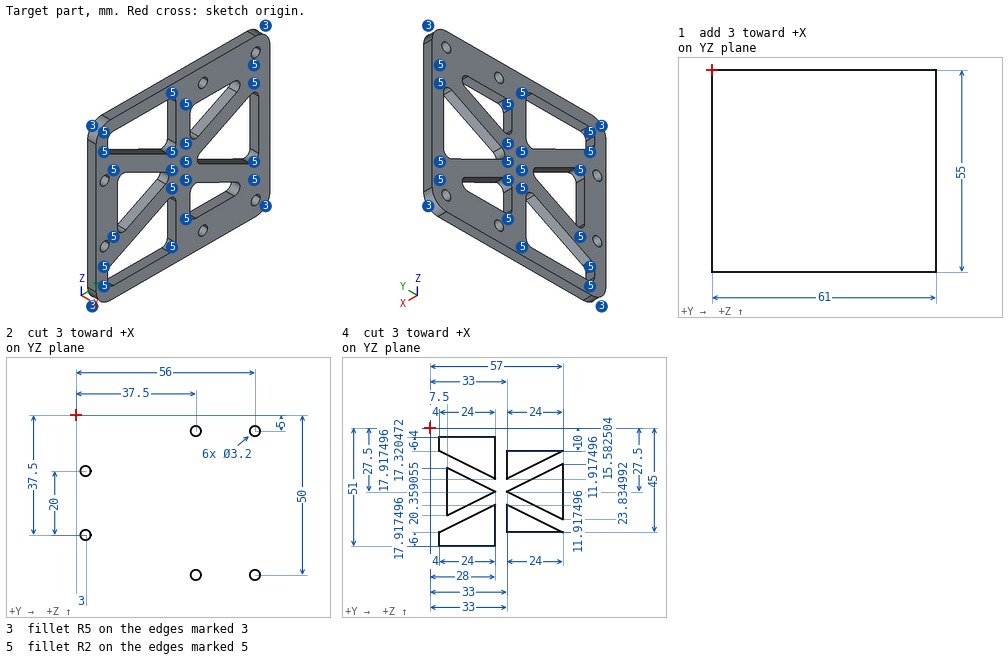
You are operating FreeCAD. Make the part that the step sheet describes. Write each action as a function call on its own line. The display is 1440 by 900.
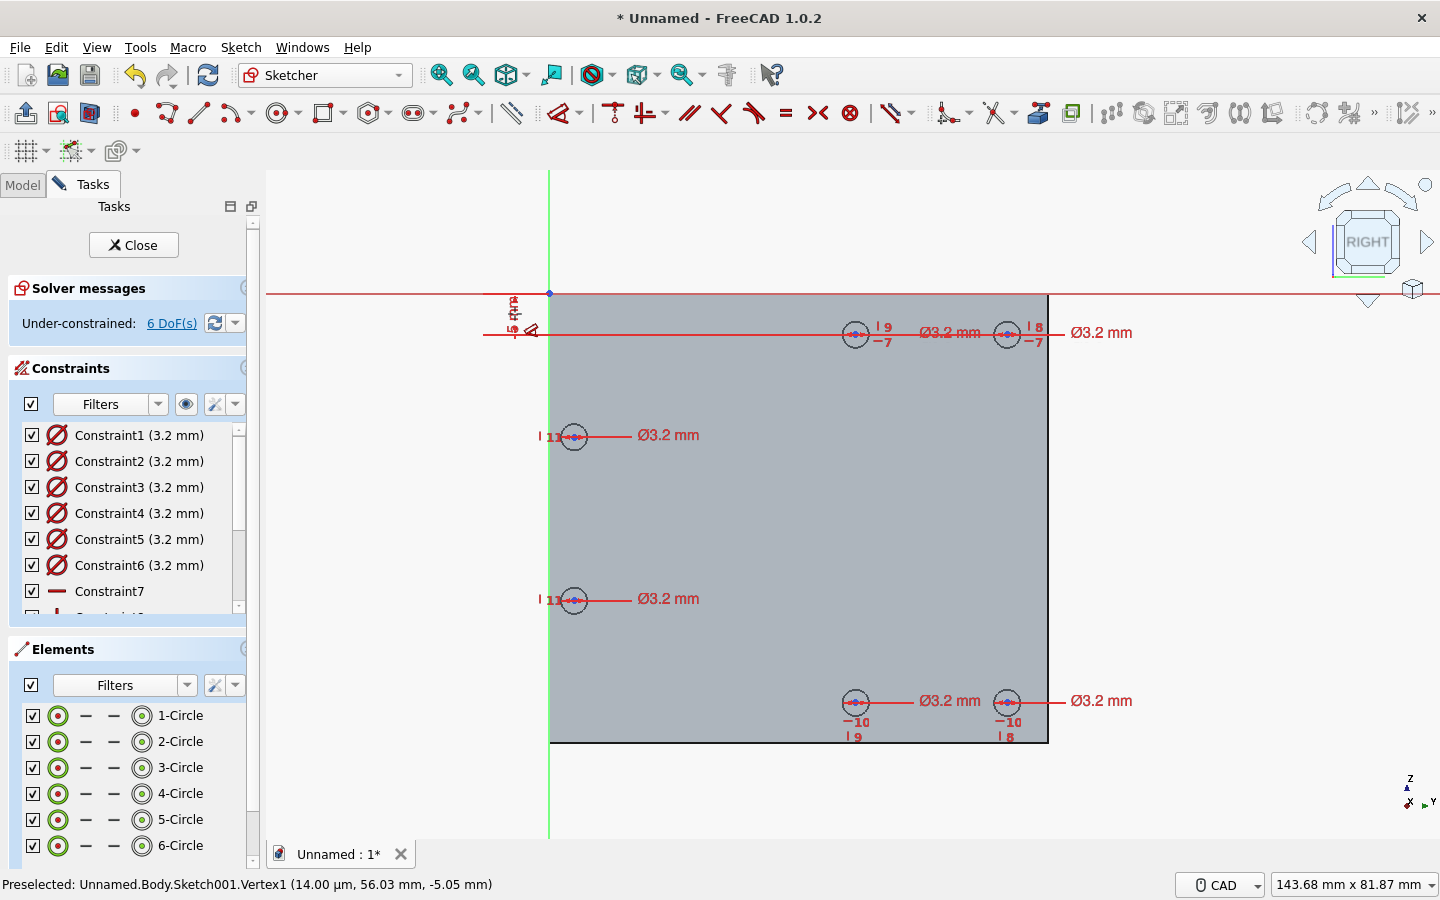
scroll(574, 601, up, 3)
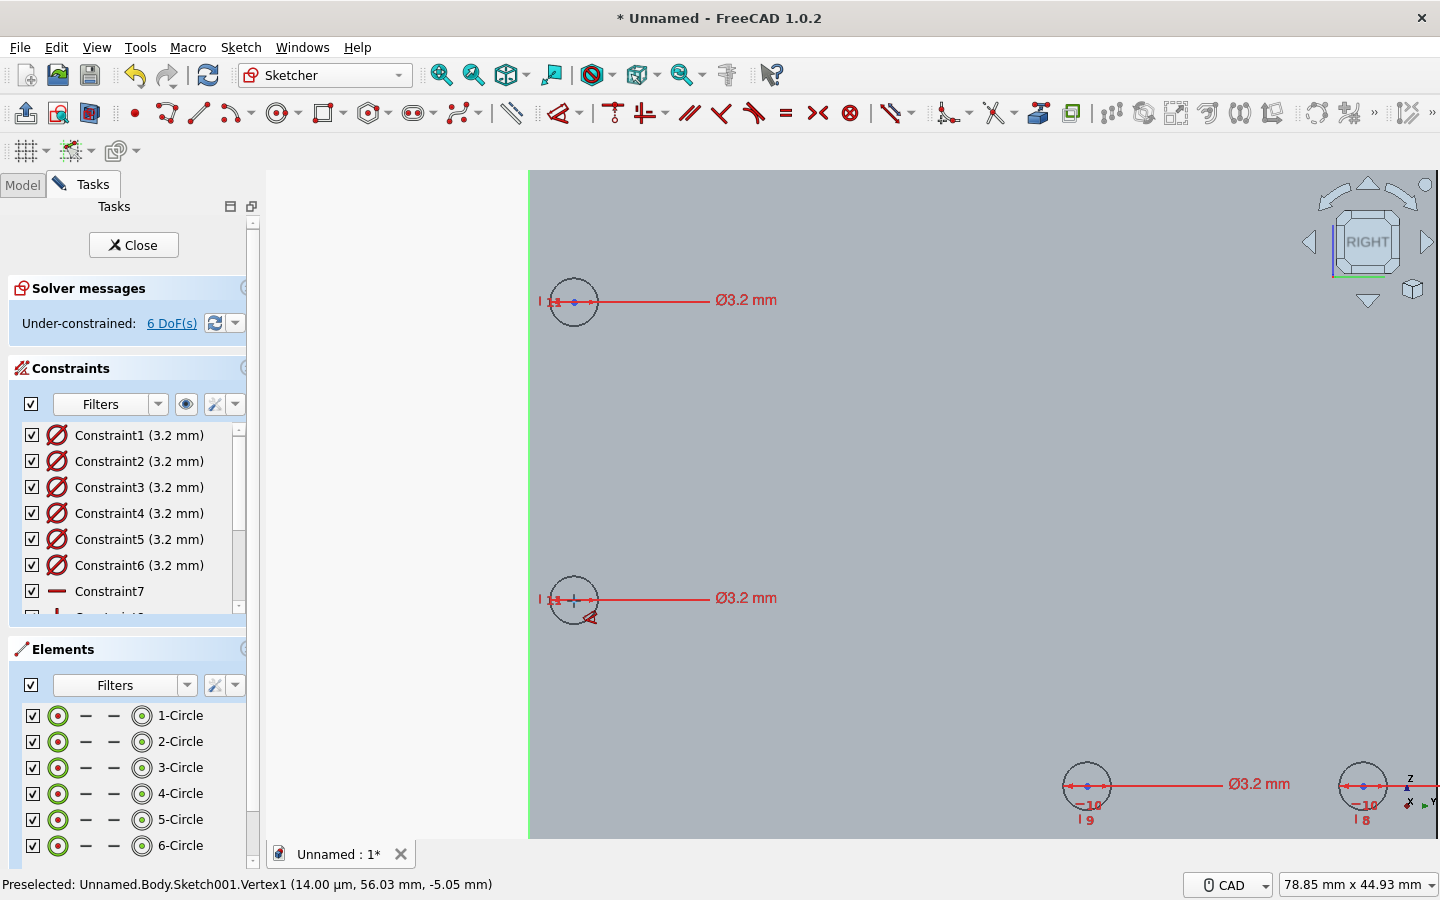
click(574, 600)
click(551, 634)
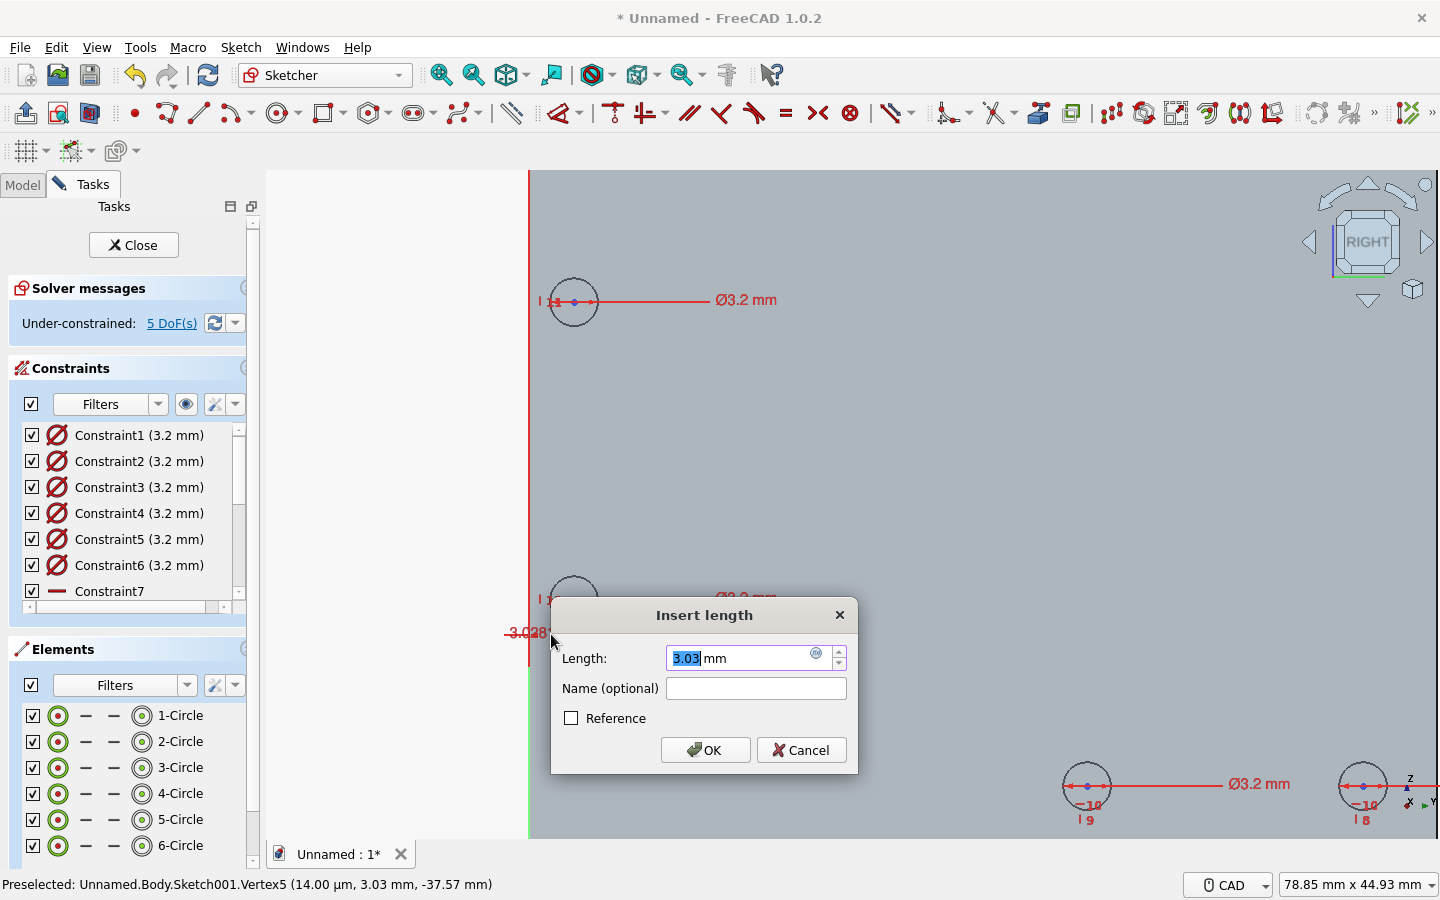
text(3)
key(Return)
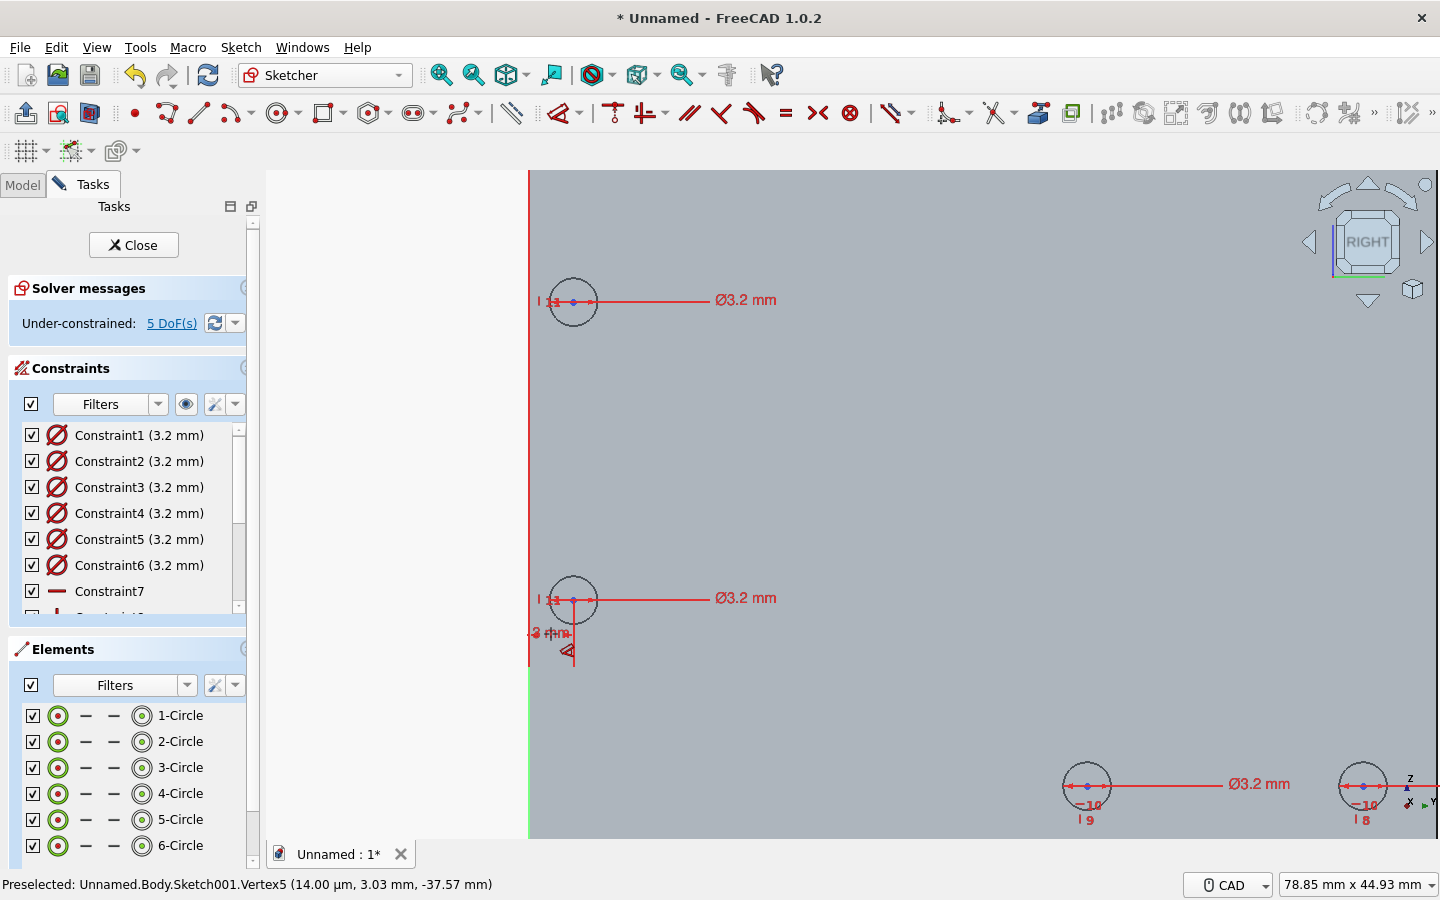
scroll(574, 601, down, 3)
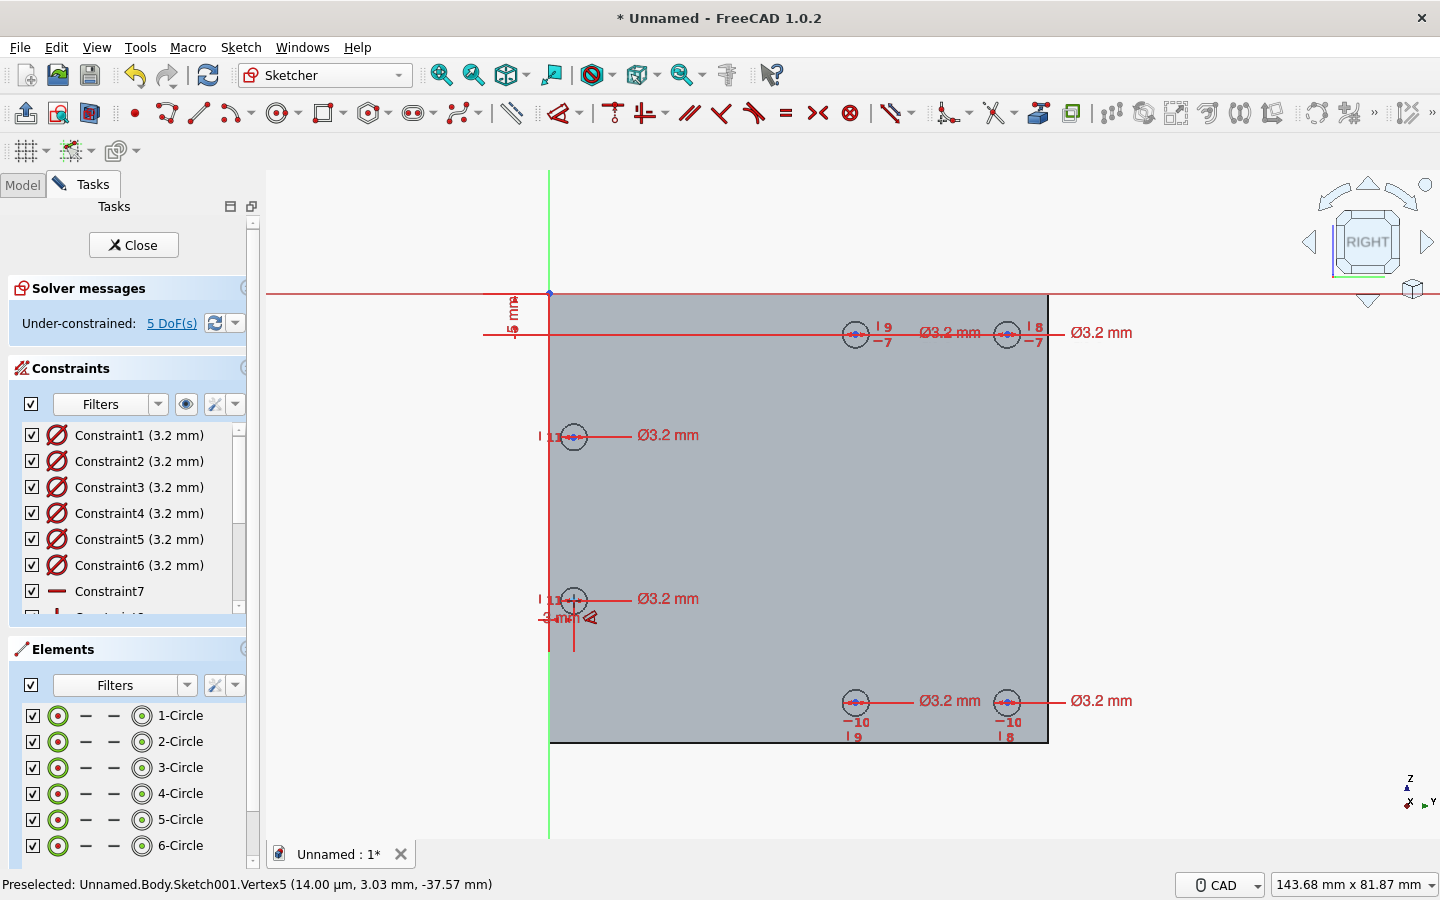
click(1007, 335)
click(778, 260)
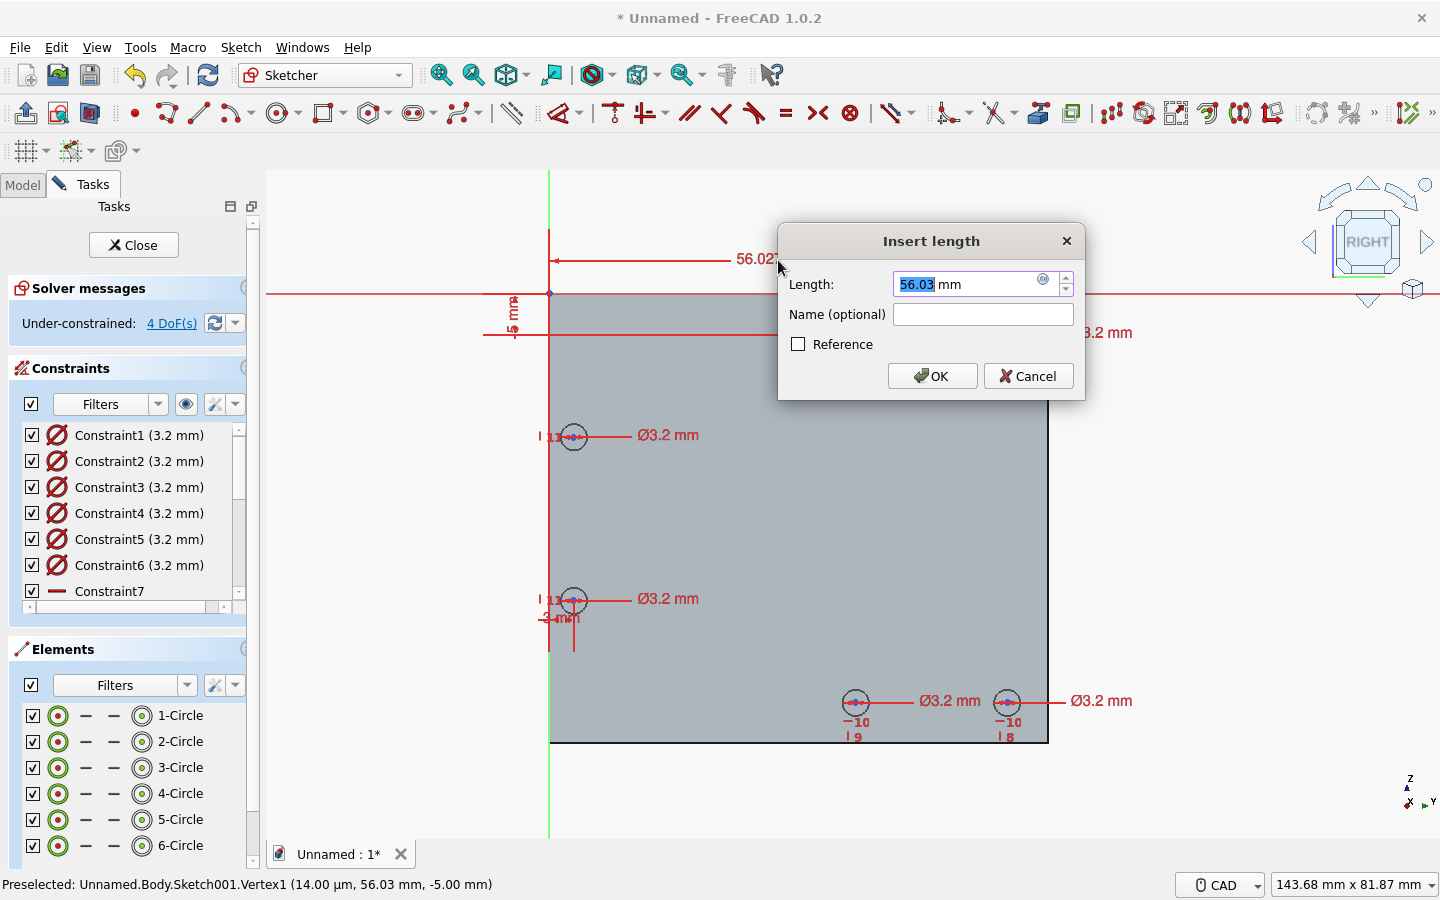
text(56)
key(Return)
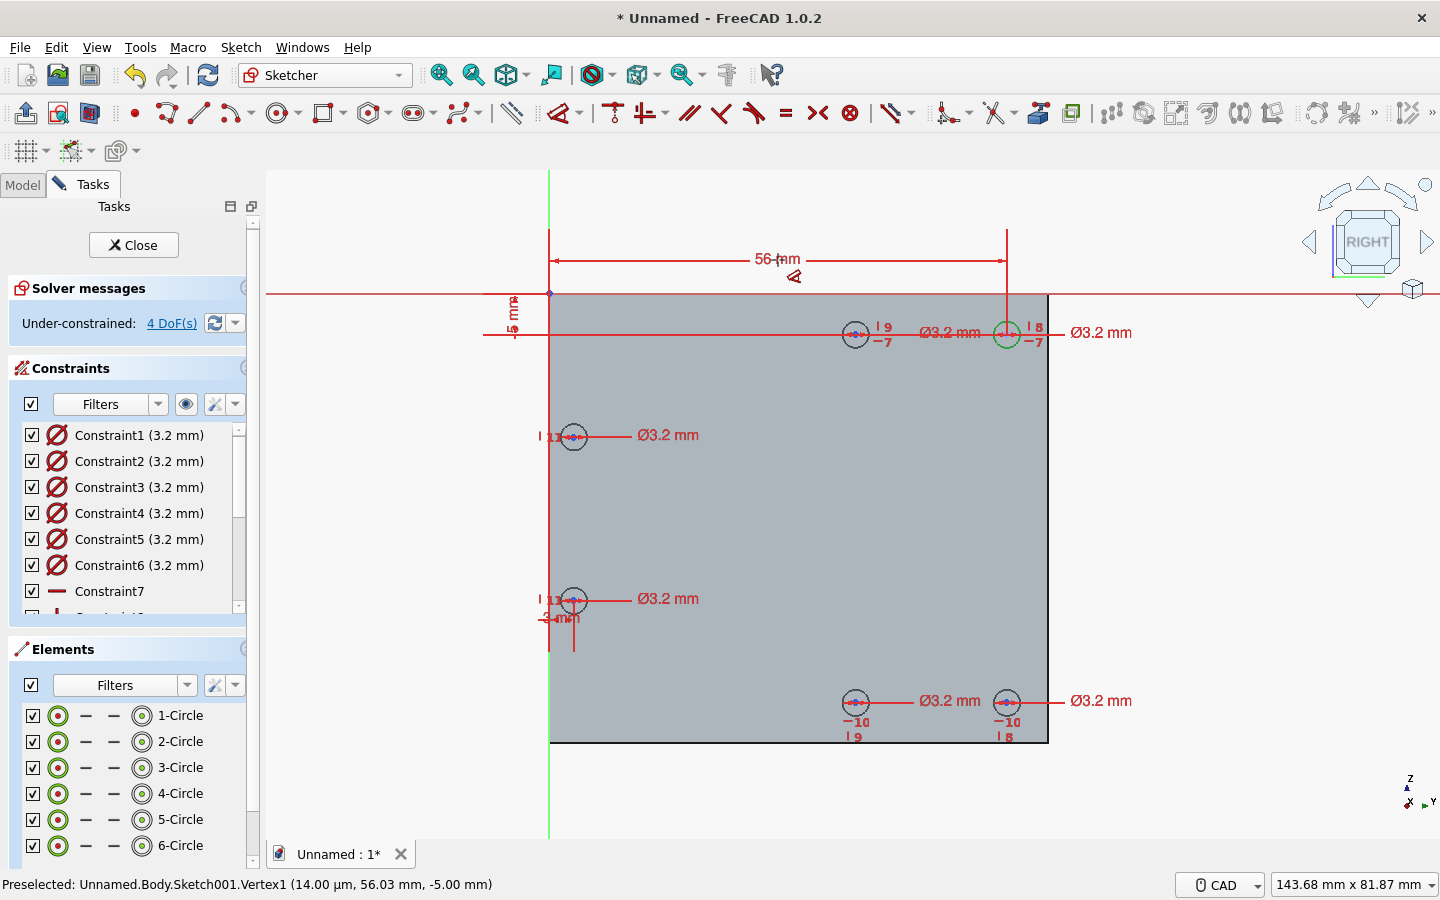
click(1007, 703)
click(515, 498)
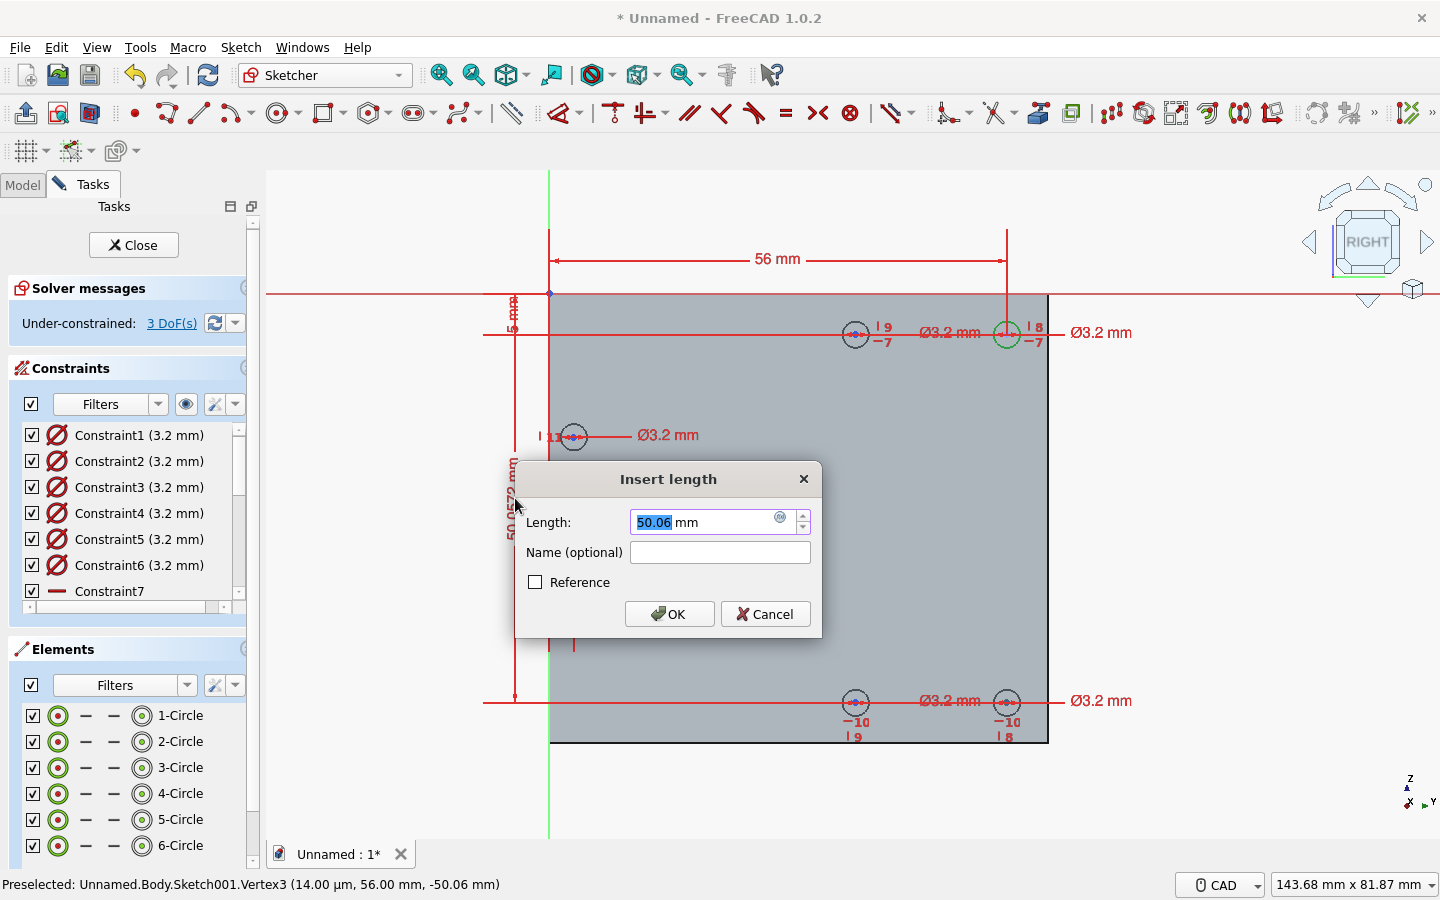
text(50)
key(Return)